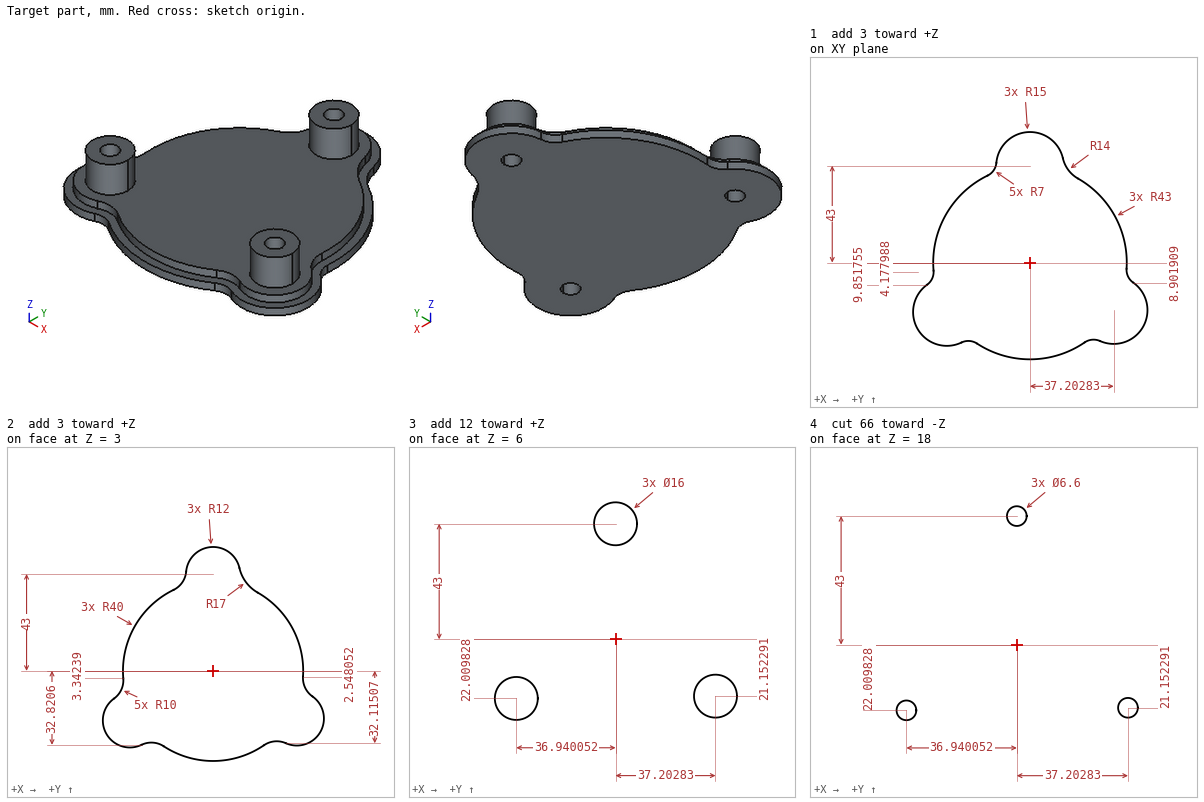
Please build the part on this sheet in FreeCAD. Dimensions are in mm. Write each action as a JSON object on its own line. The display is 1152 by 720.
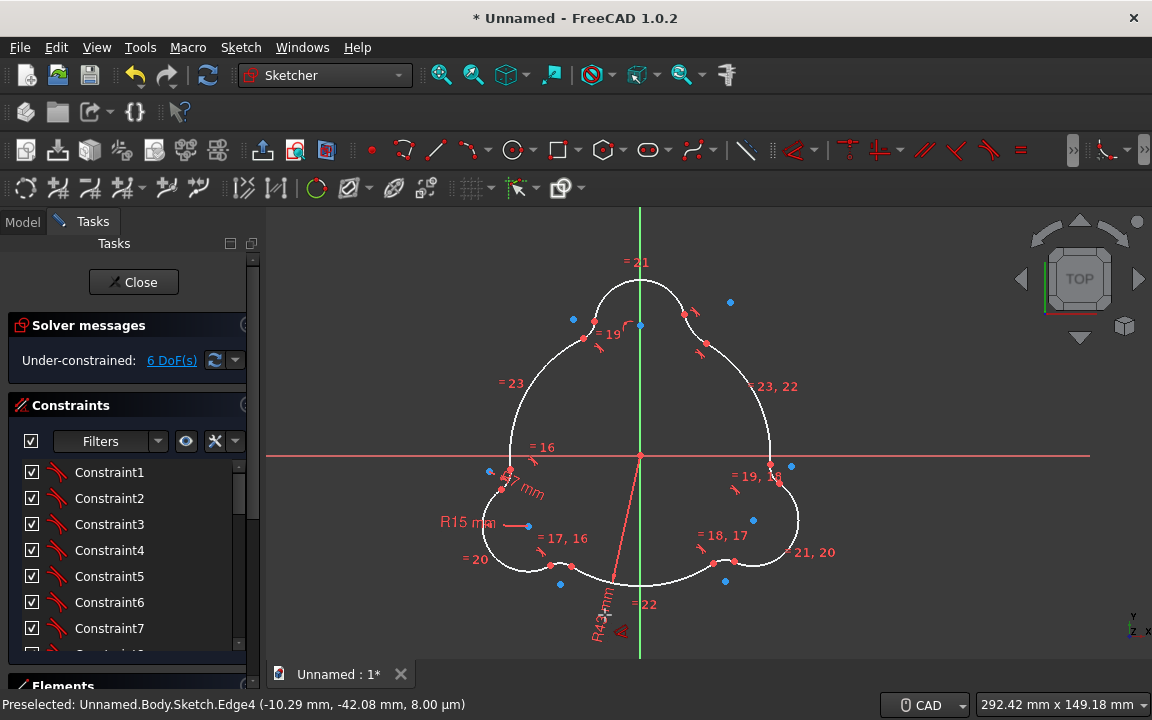
{"action": "scroll", "coordinate": [688, 325], "scroll_direction": "up", "scroll_amount": 2}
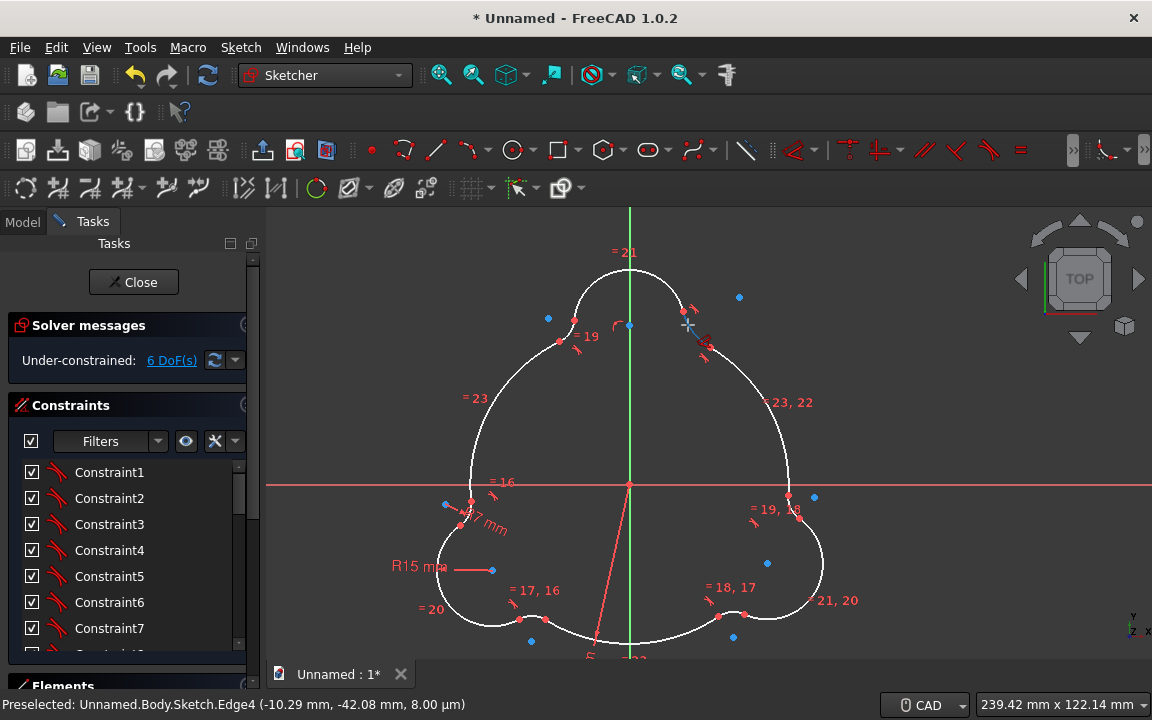
{"action": "left_click", "coordinate": [688, 324]}
{"action": "left_click", "coordinate": [660, 339]}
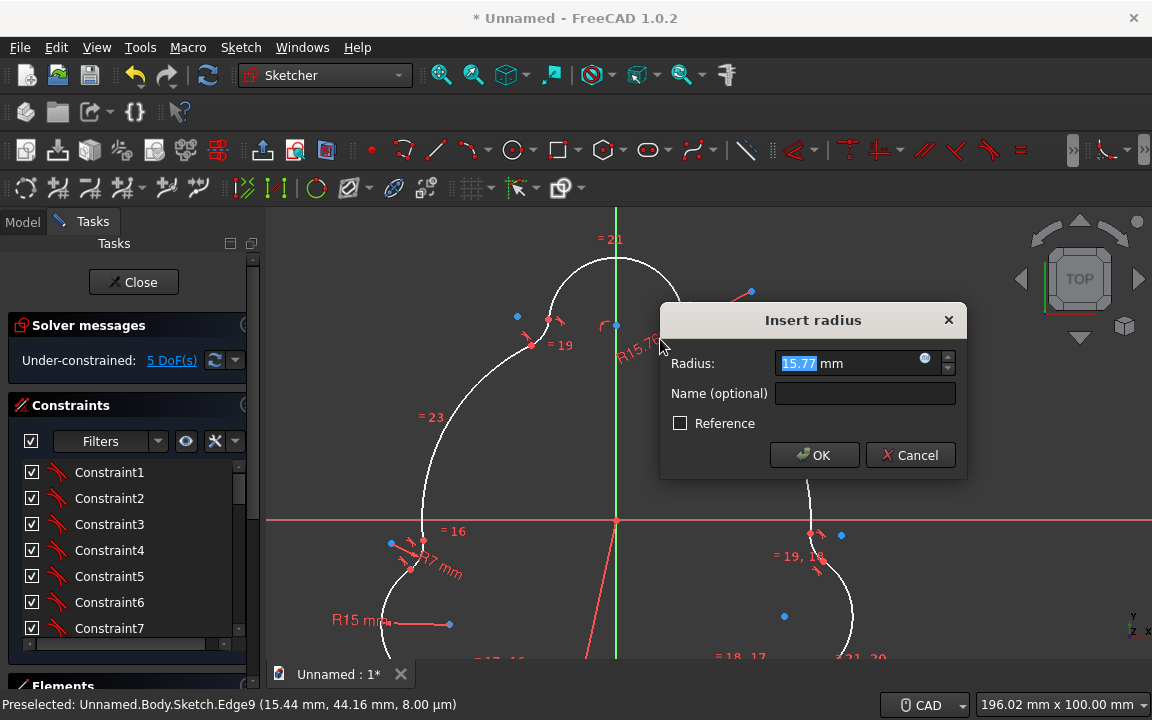
{"action": "type", "text": "14"}
{"action": "key", "text": "Return"}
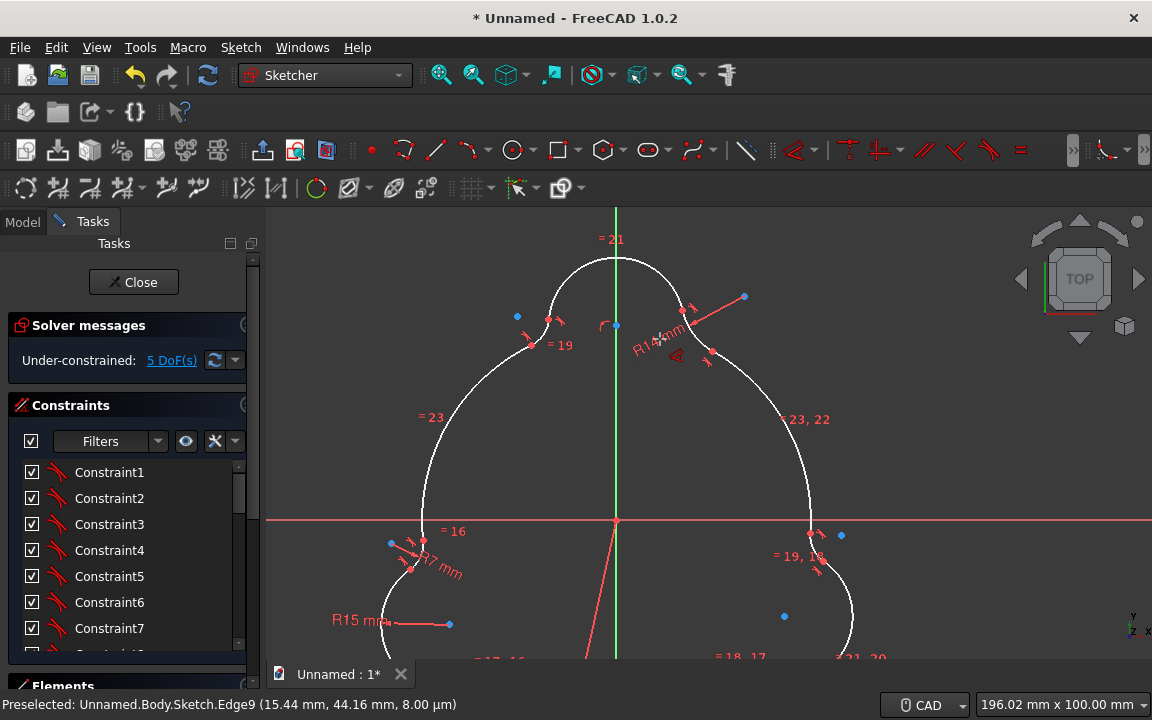
{"action": "left_click", "coordinate": [616, 326]}
{"action": "left_click", "coordinate": [582, 423]}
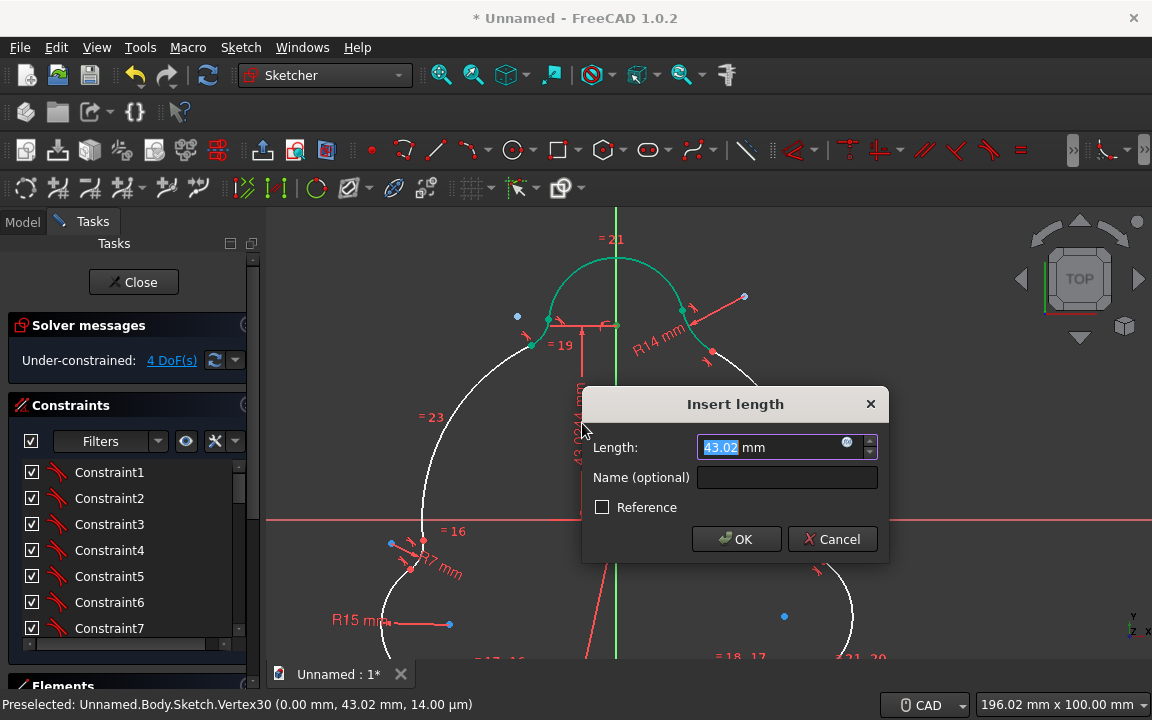
{"action": "type", "text": "43"}
{"action": "key", "text": "Return"}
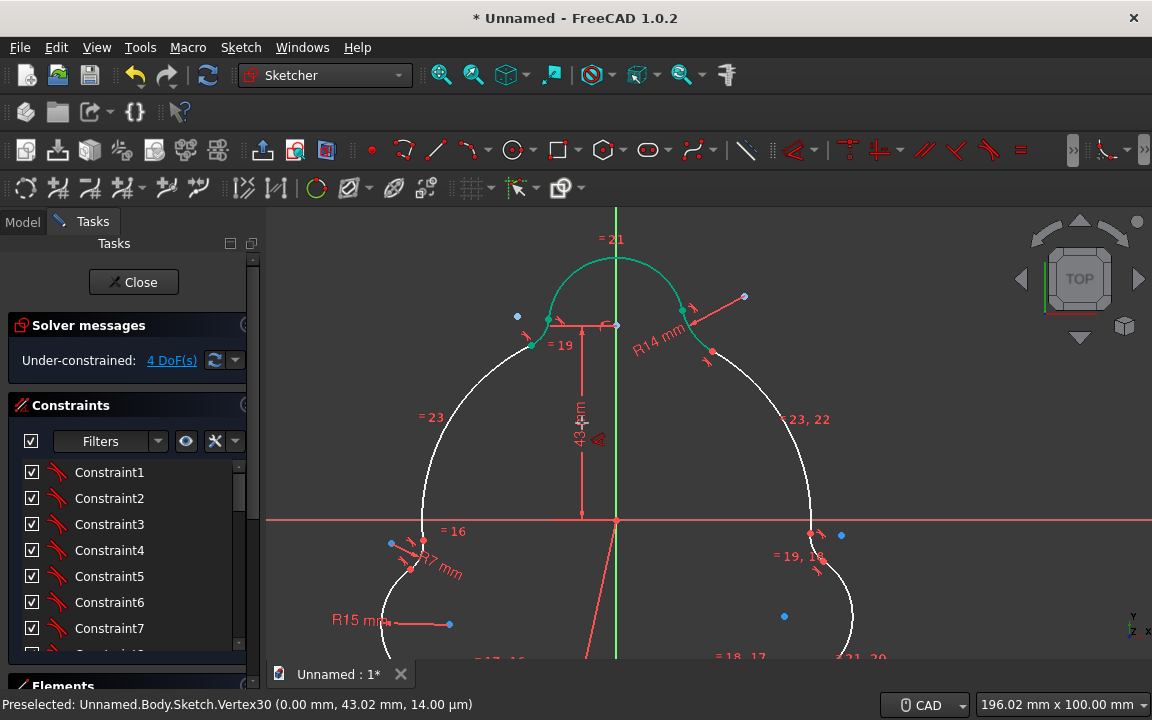
{"action": "left_click", "coordinate": [410, 570]}
{"action": "left_click", "coordinate": [376, 533]}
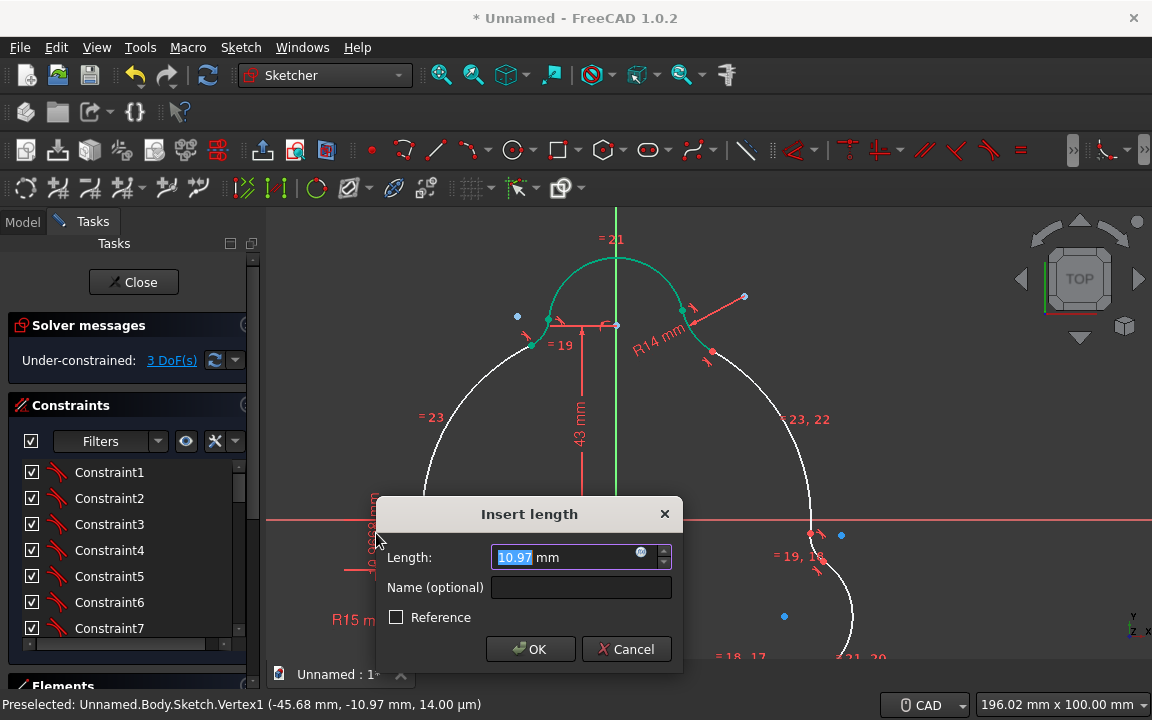
{"action": "type", "text": "9.851755"}
{"action": "key", "text": "Return"}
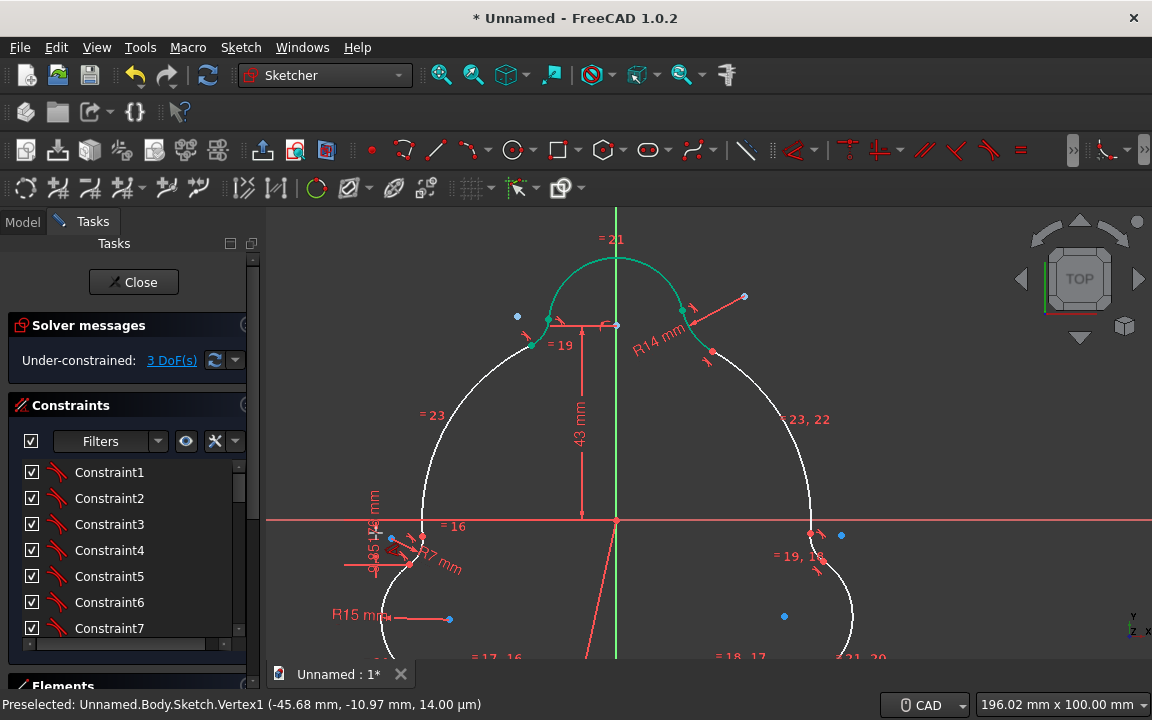
{"action": "left_click", "coordinate": [824, 561]}
{"action": "left_click", "coordinate": [858, 541]}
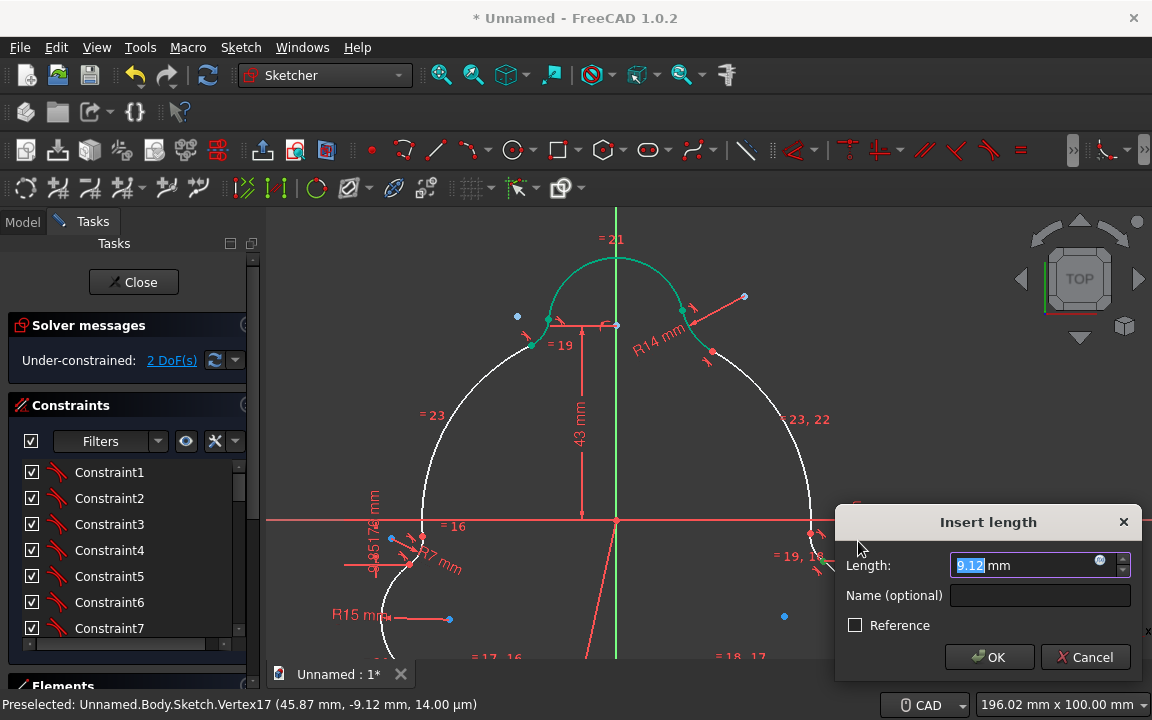
{"action": "type", "text": "8.901909"}
{"action": "key", "text": "Return"}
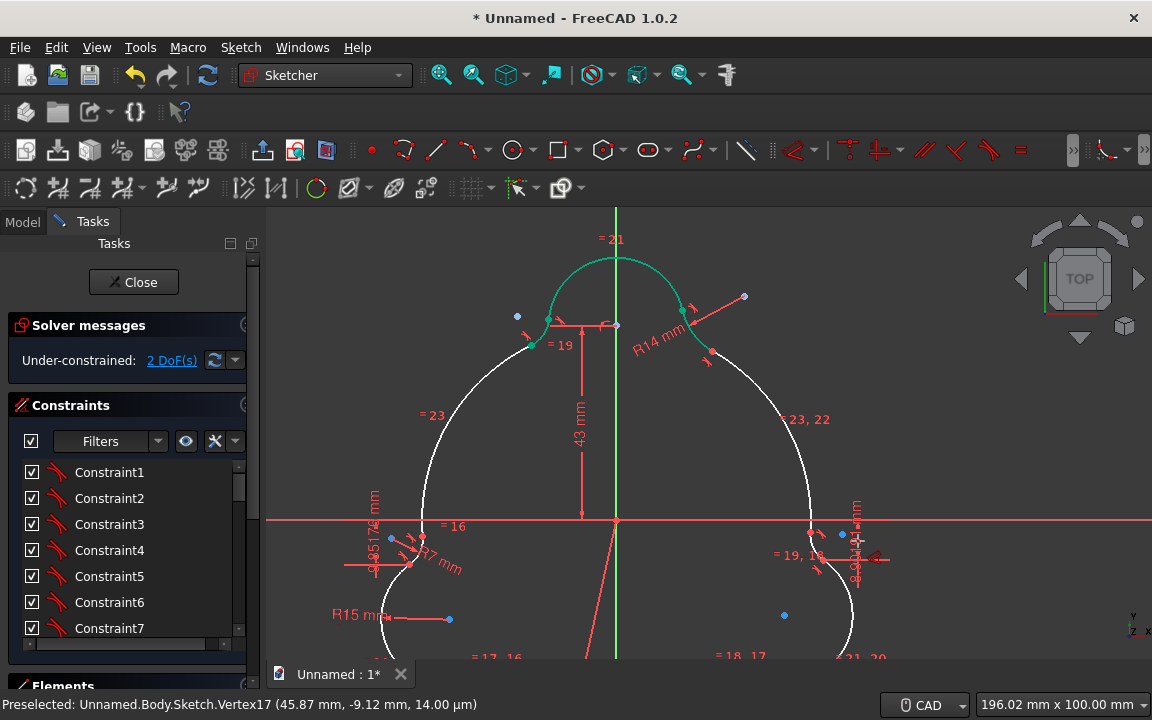
{"action": "scroll", "coordinate": [391, 539], "scroll_direction": "up", "scroll_amount": 4}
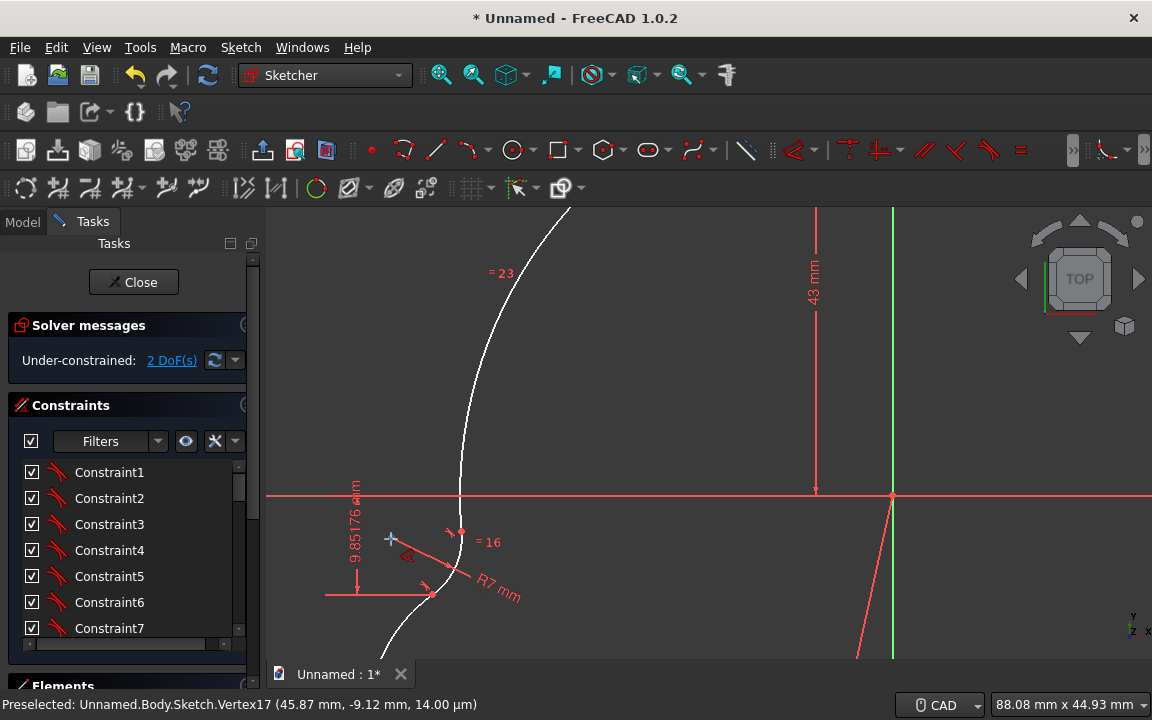
{"action": "left_click", "coordinate": [391, 538]}
{"action": "left_click", "coordinate": [927, 517]}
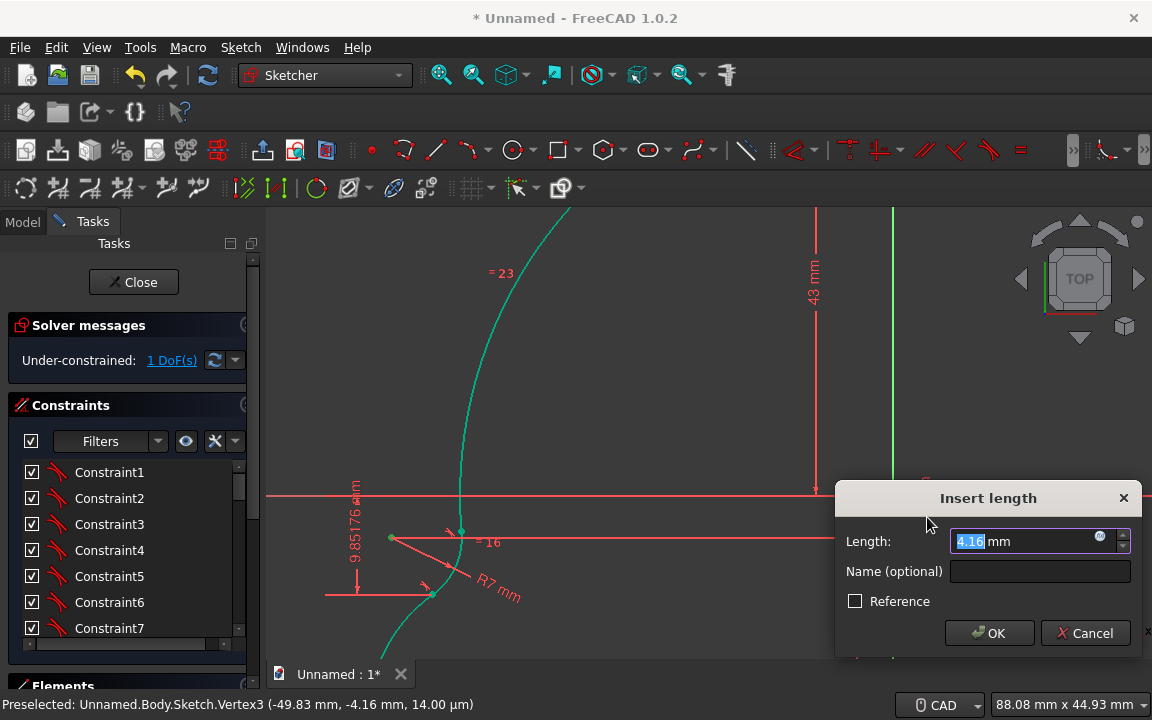
{"action": "type", "text": "4.177988"}
{"action": "key", "text": "Return"}